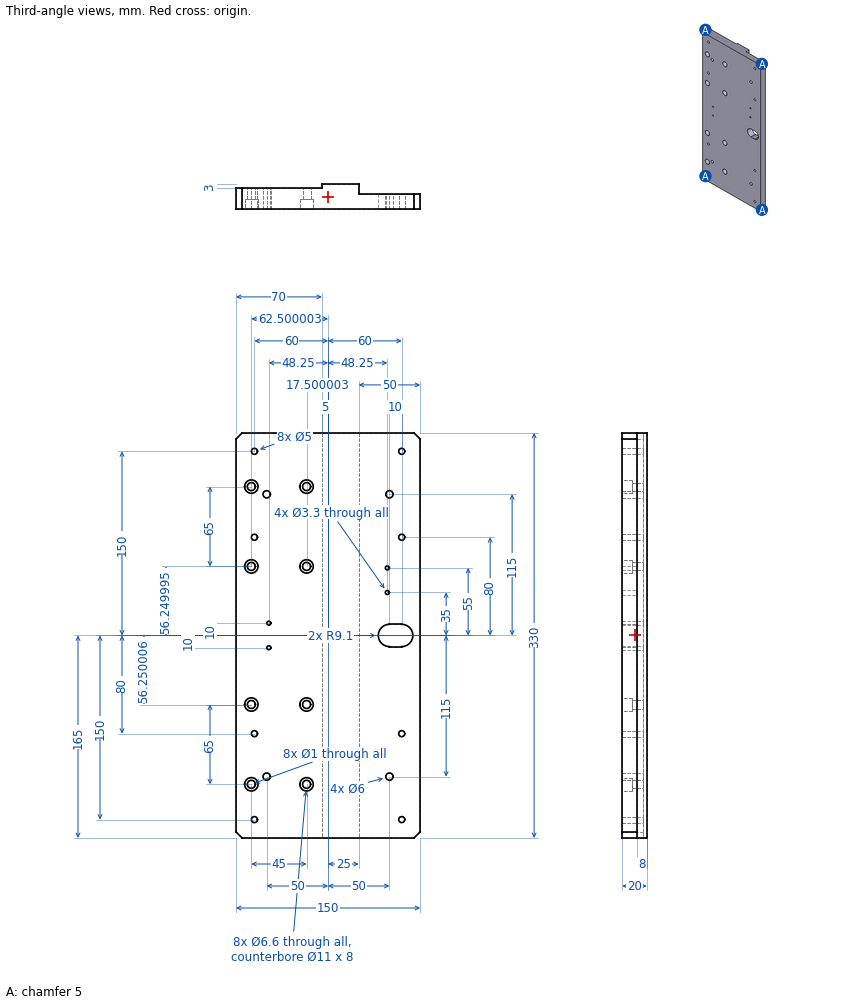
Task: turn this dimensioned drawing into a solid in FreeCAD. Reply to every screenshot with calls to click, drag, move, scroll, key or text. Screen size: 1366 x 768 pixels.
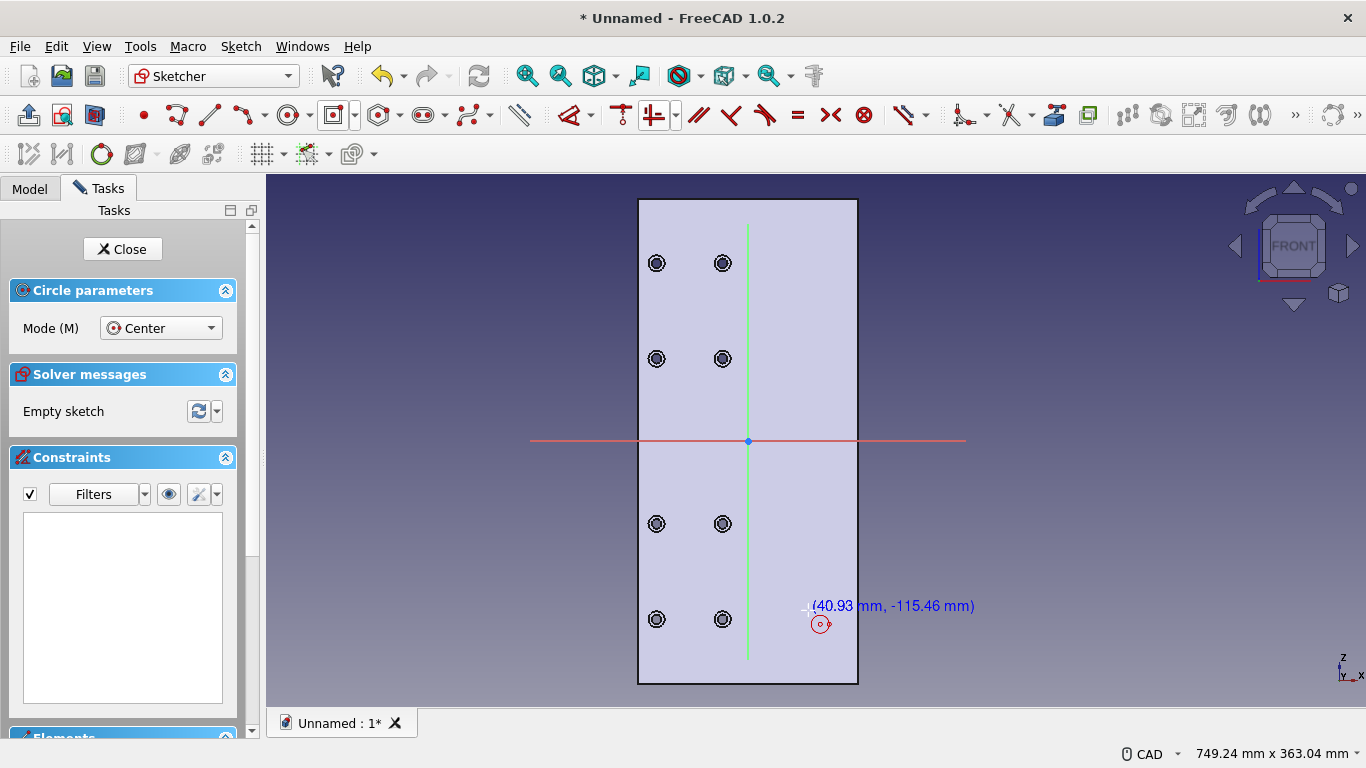
click(822, 610)
move(825, 607)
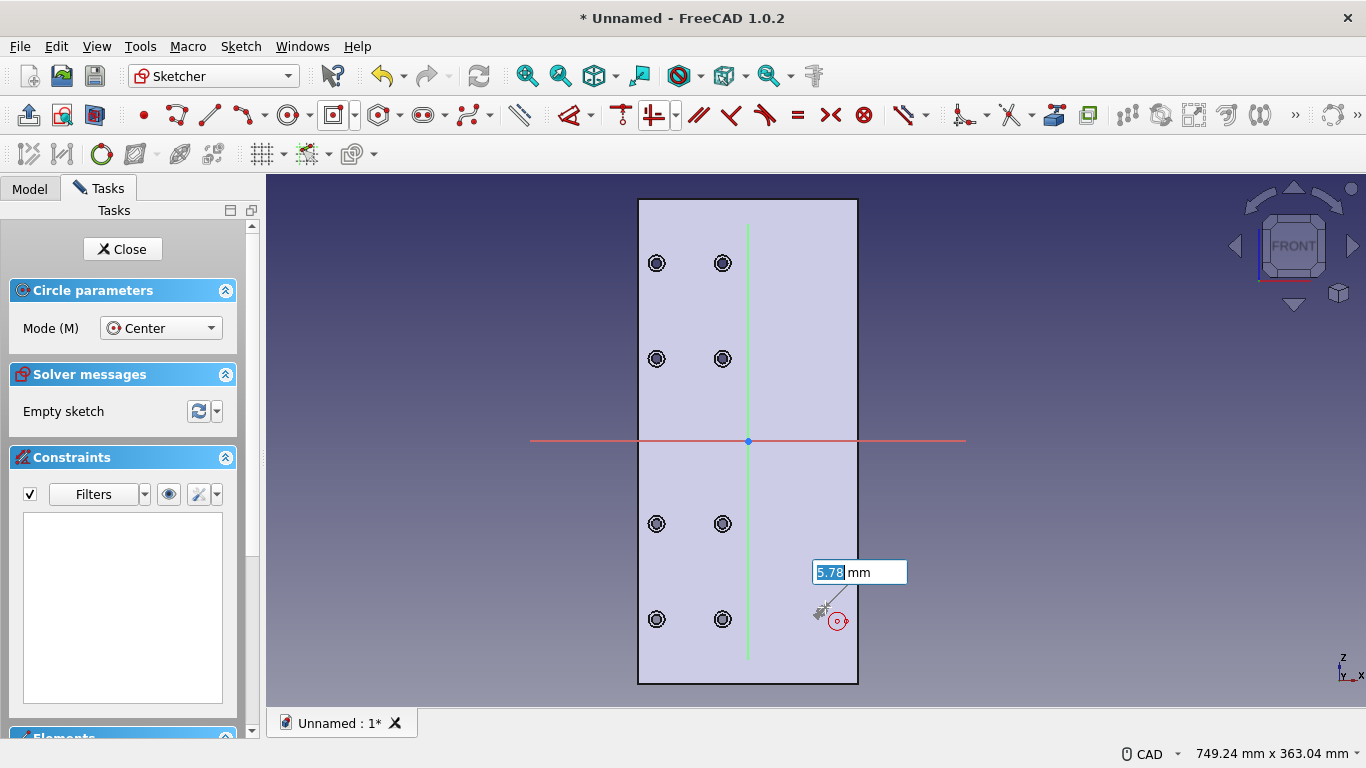
text(6)
key(Return)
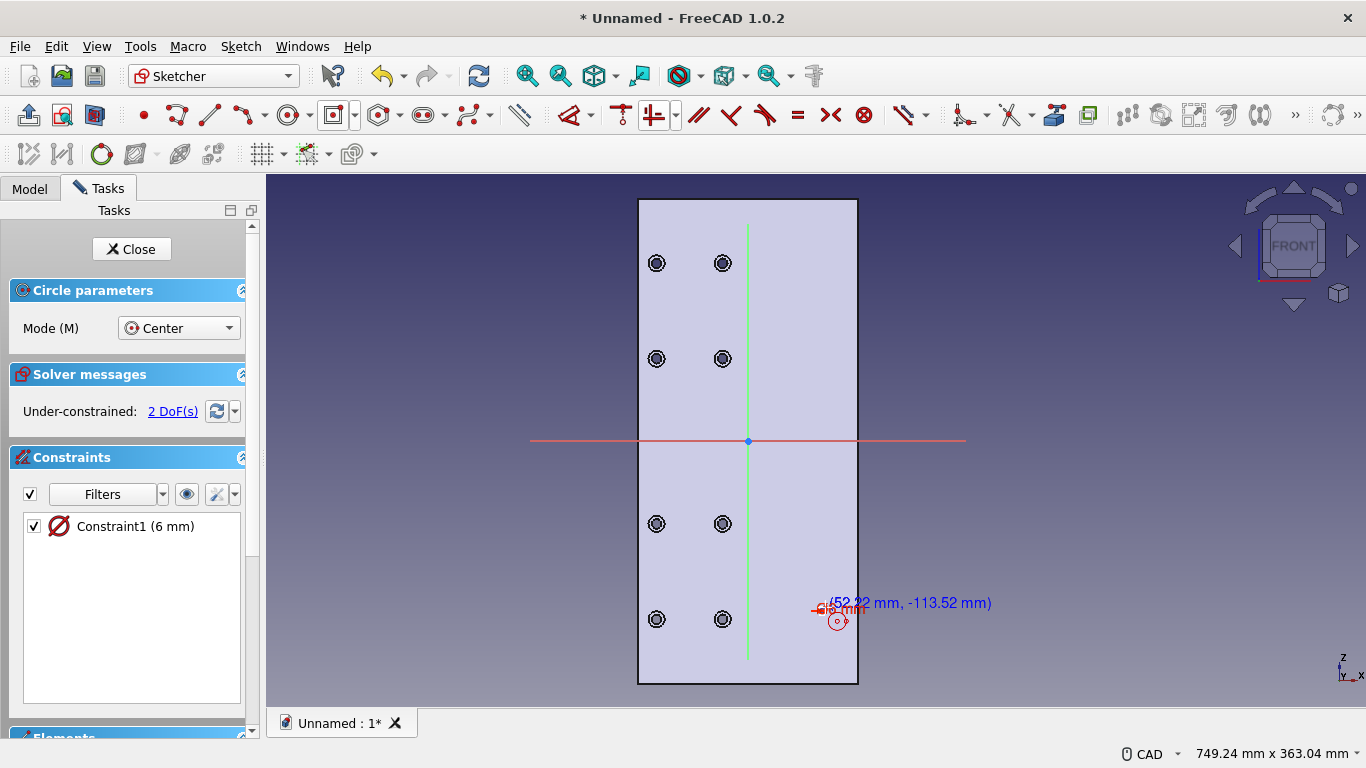
scroll(822, 272, up, 9)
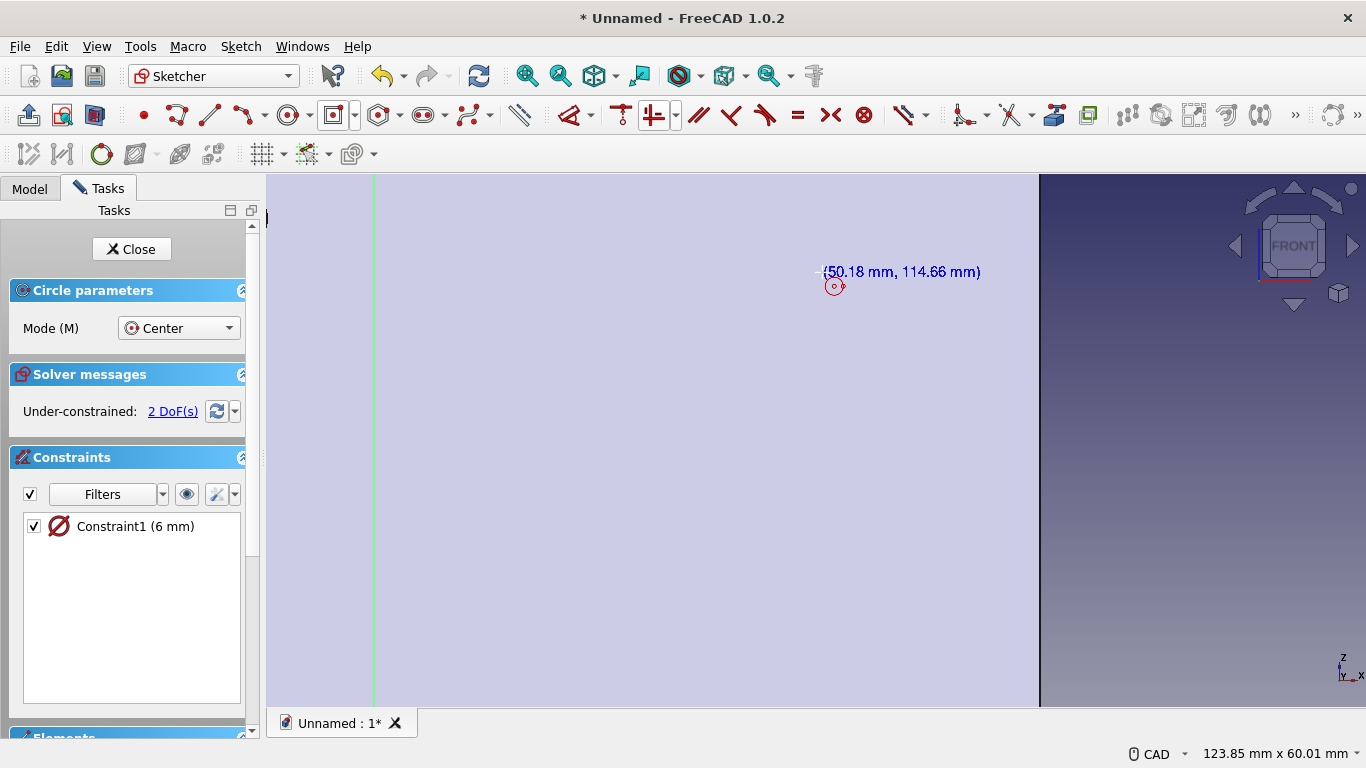
scroll(822, 271, down, 9)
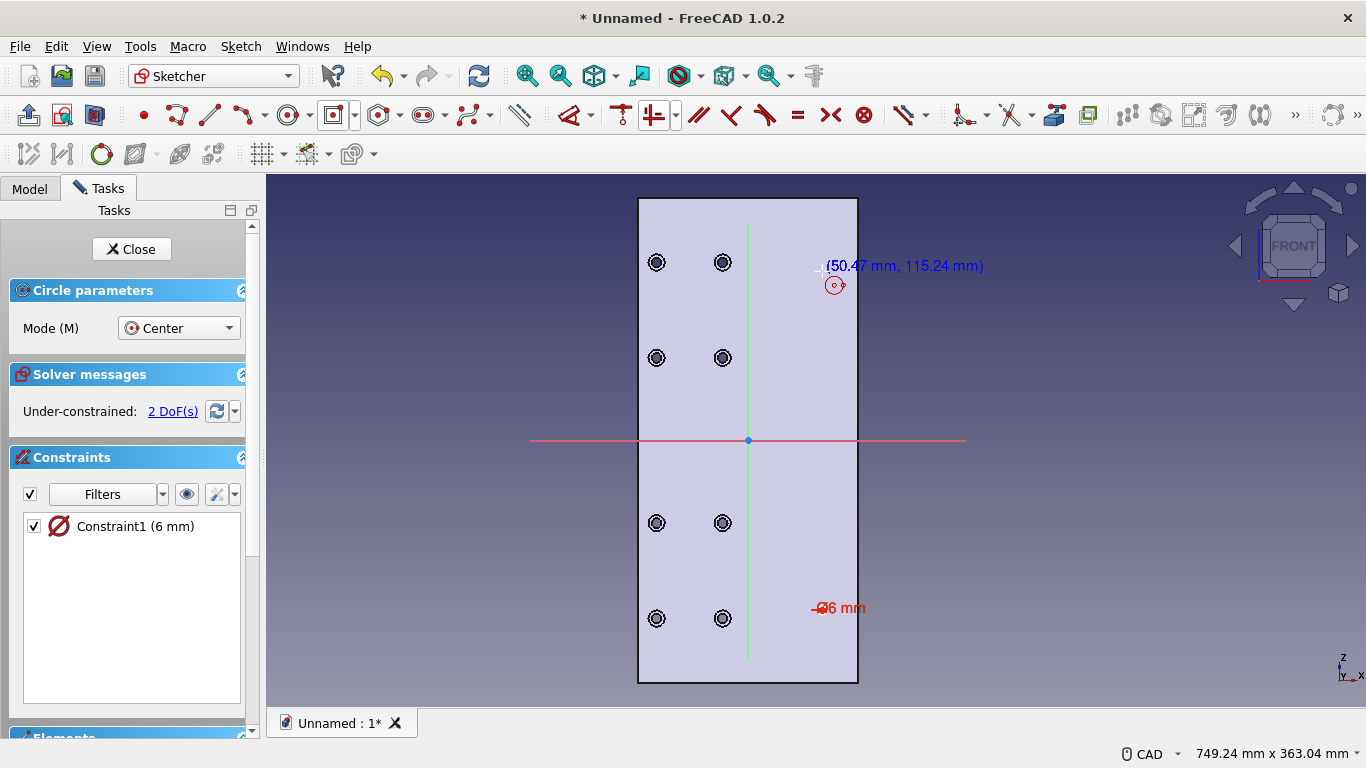
click(822, 272)
move(825, 269)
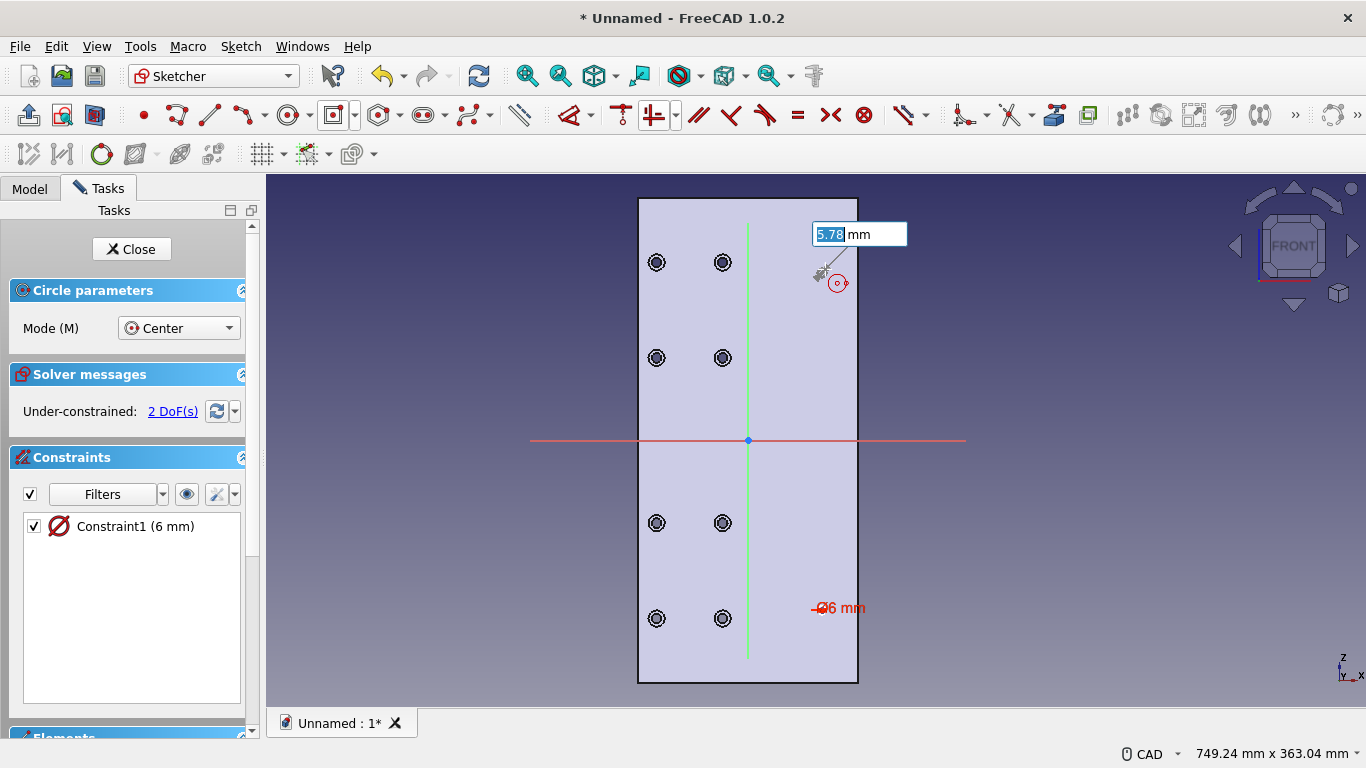
text(6)
key(Return)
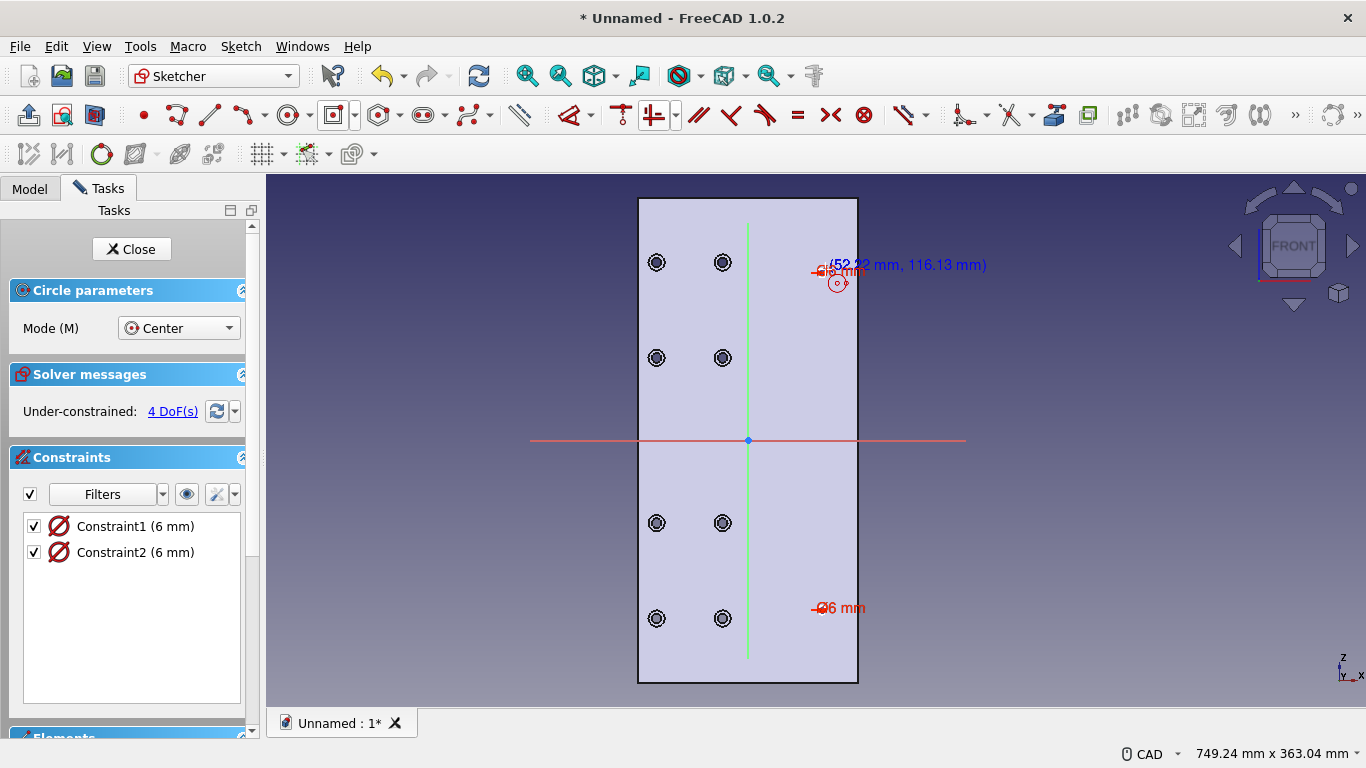
scroll(675, 609, up, 9)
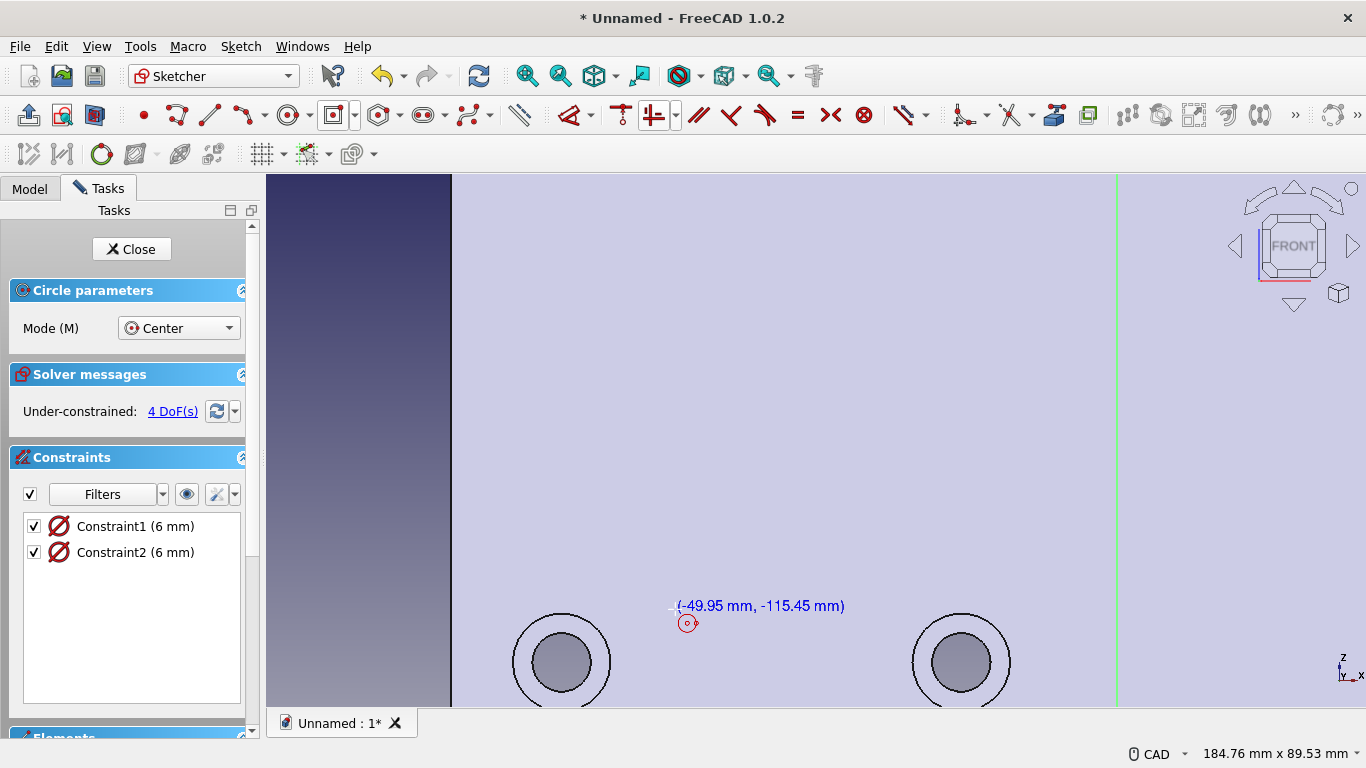
scroll(674, 610, down, 9)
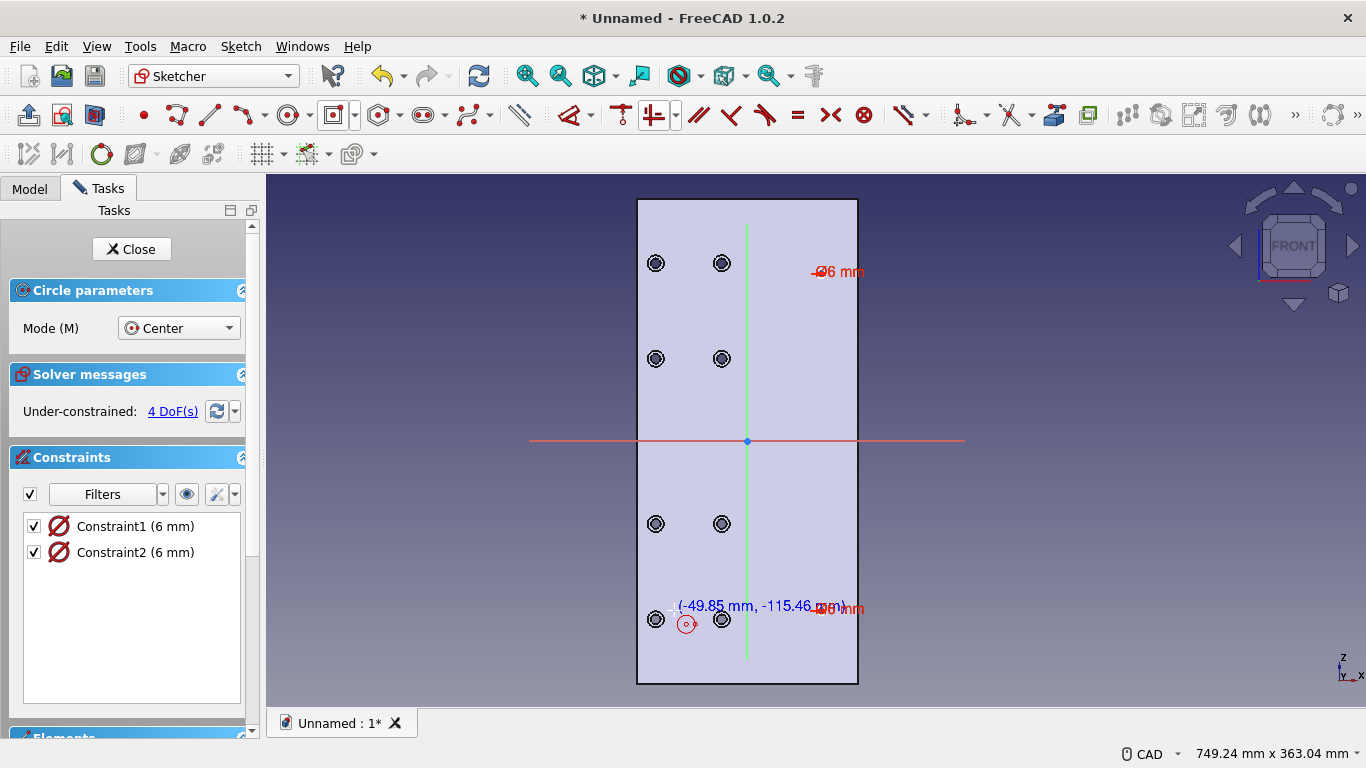
click(674, 610)
move(677, 607)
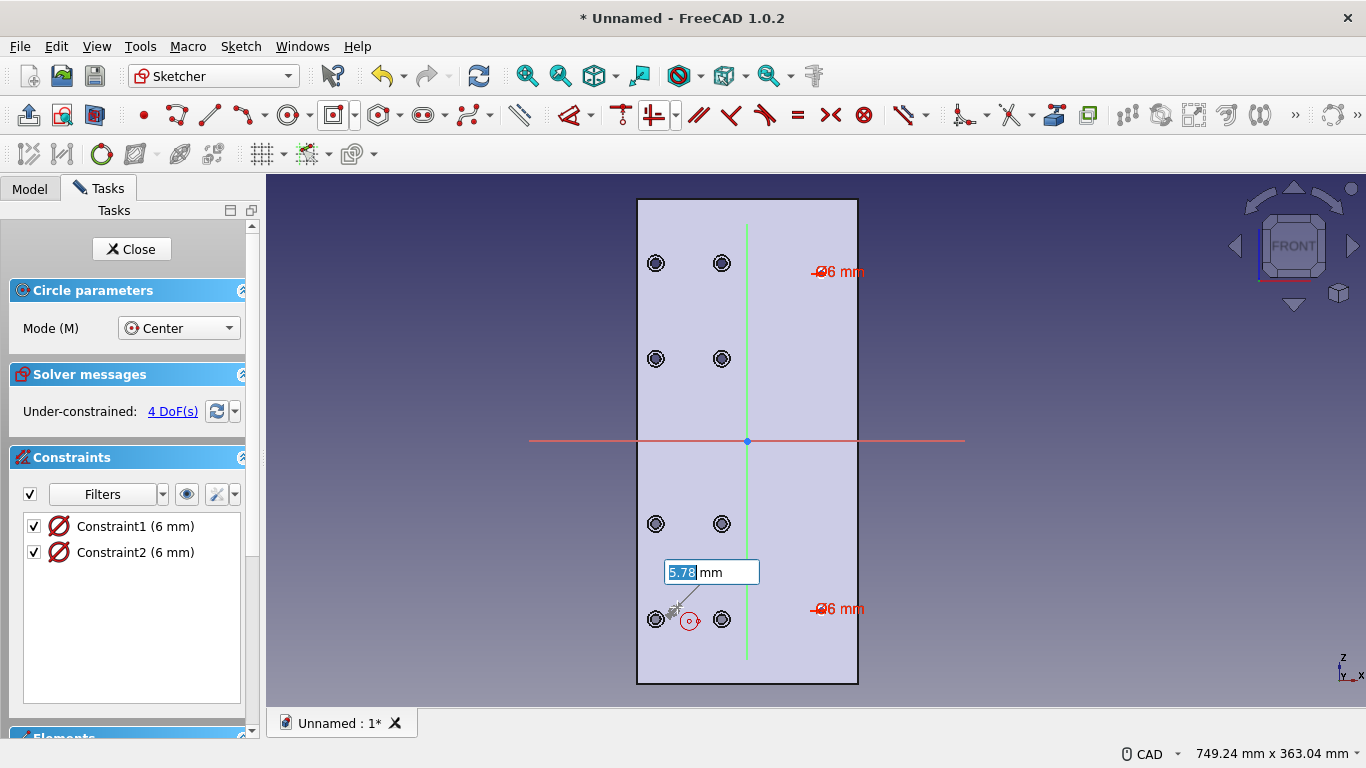
text(6)
key(Return)